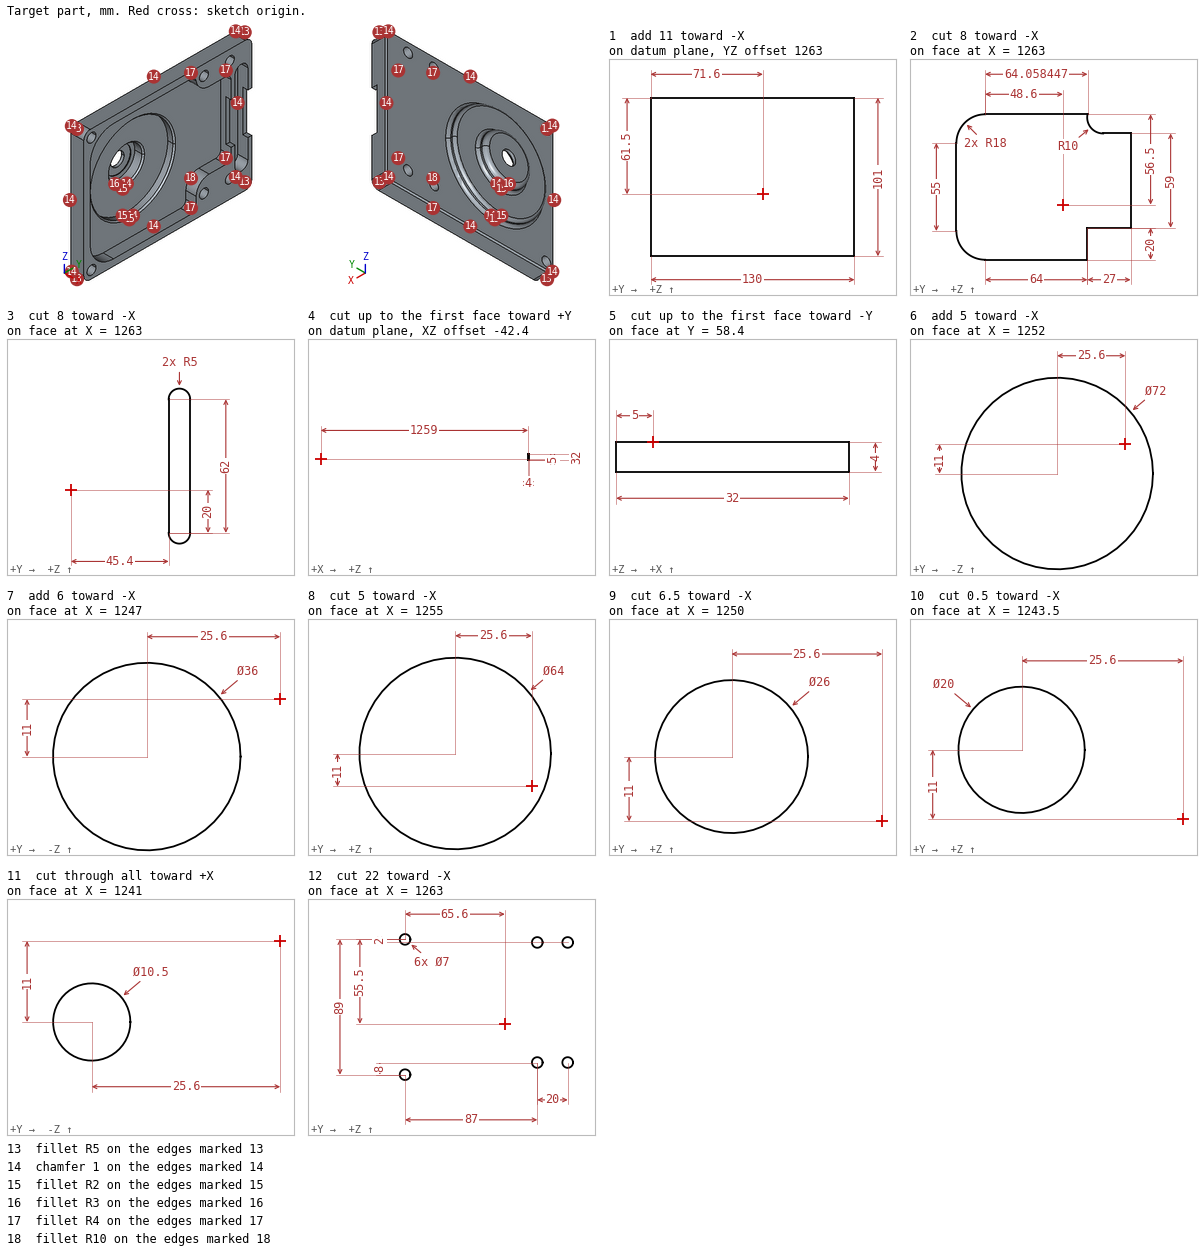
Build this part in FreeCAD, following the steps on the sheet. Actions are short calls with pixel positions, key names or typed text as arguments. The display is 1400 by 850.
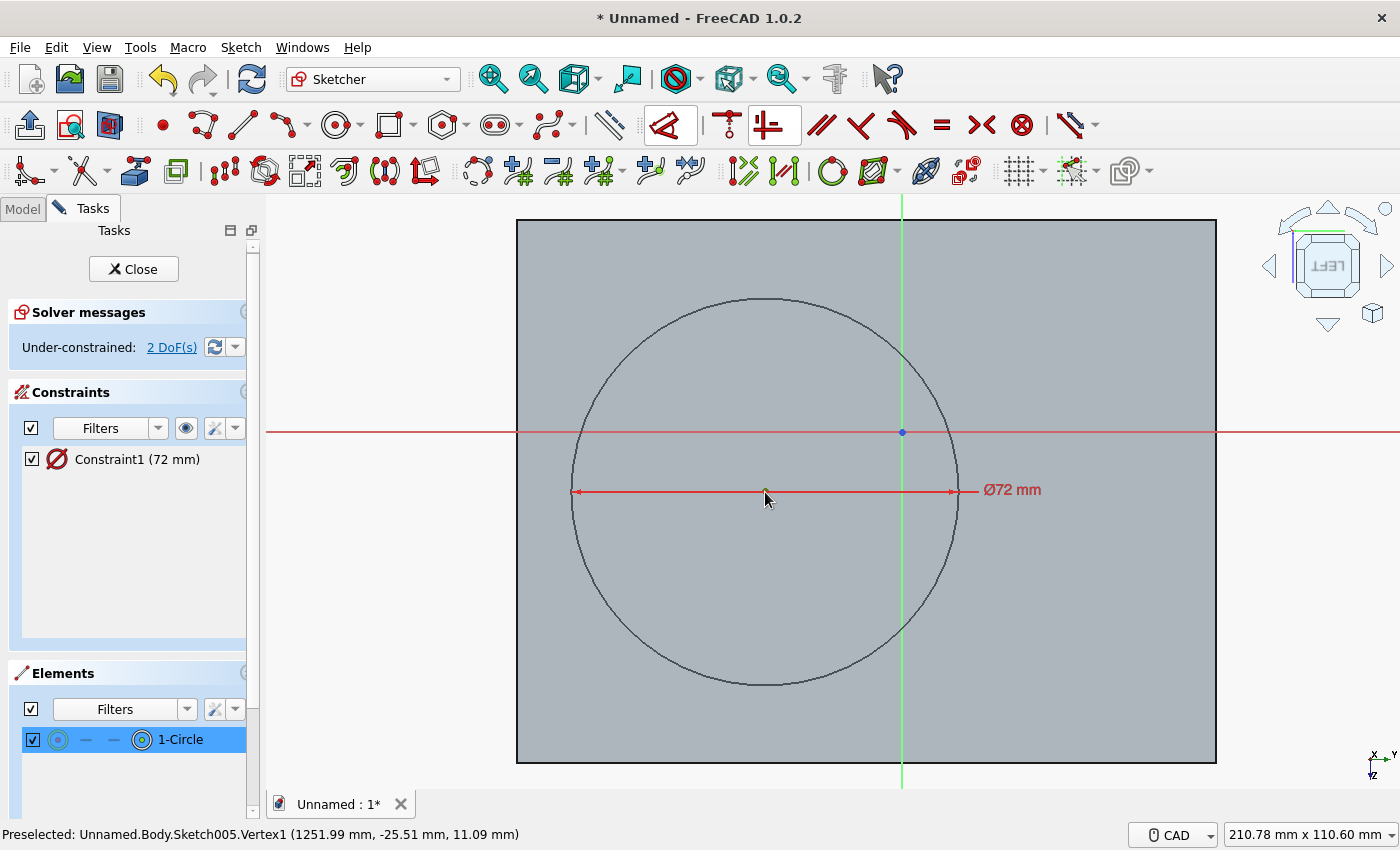
key(i)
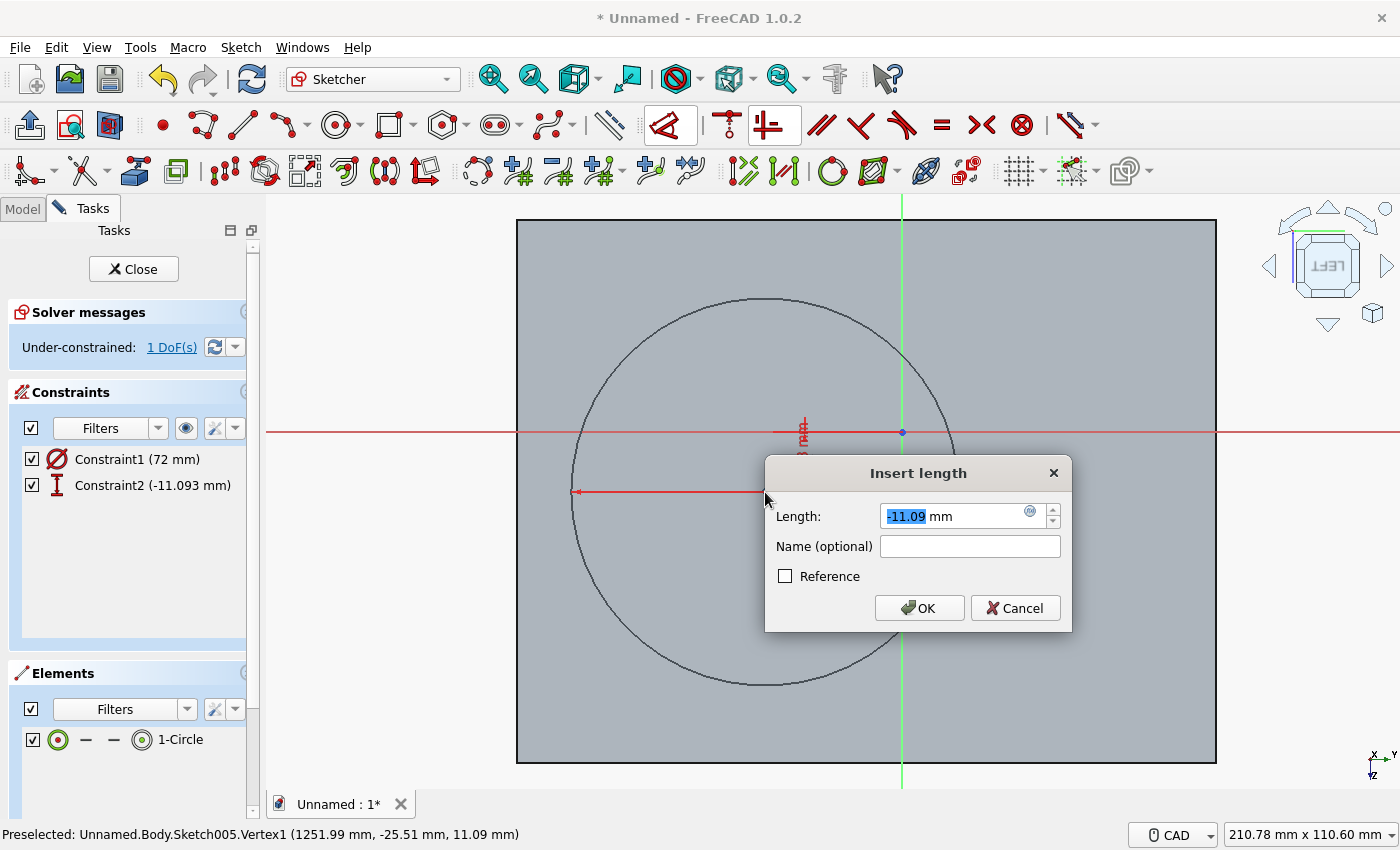
text(-11)
key(Return)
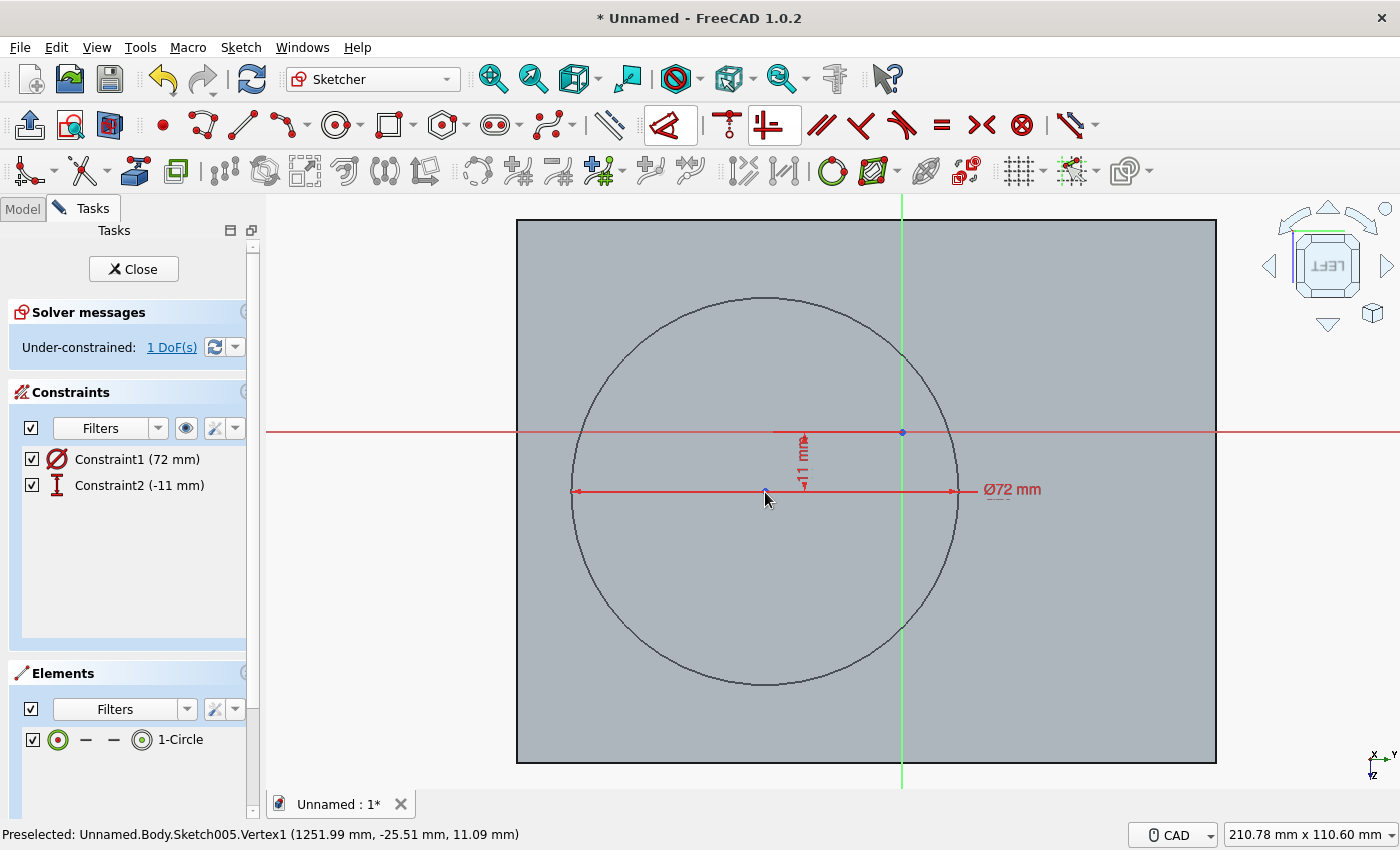
click(765, 491)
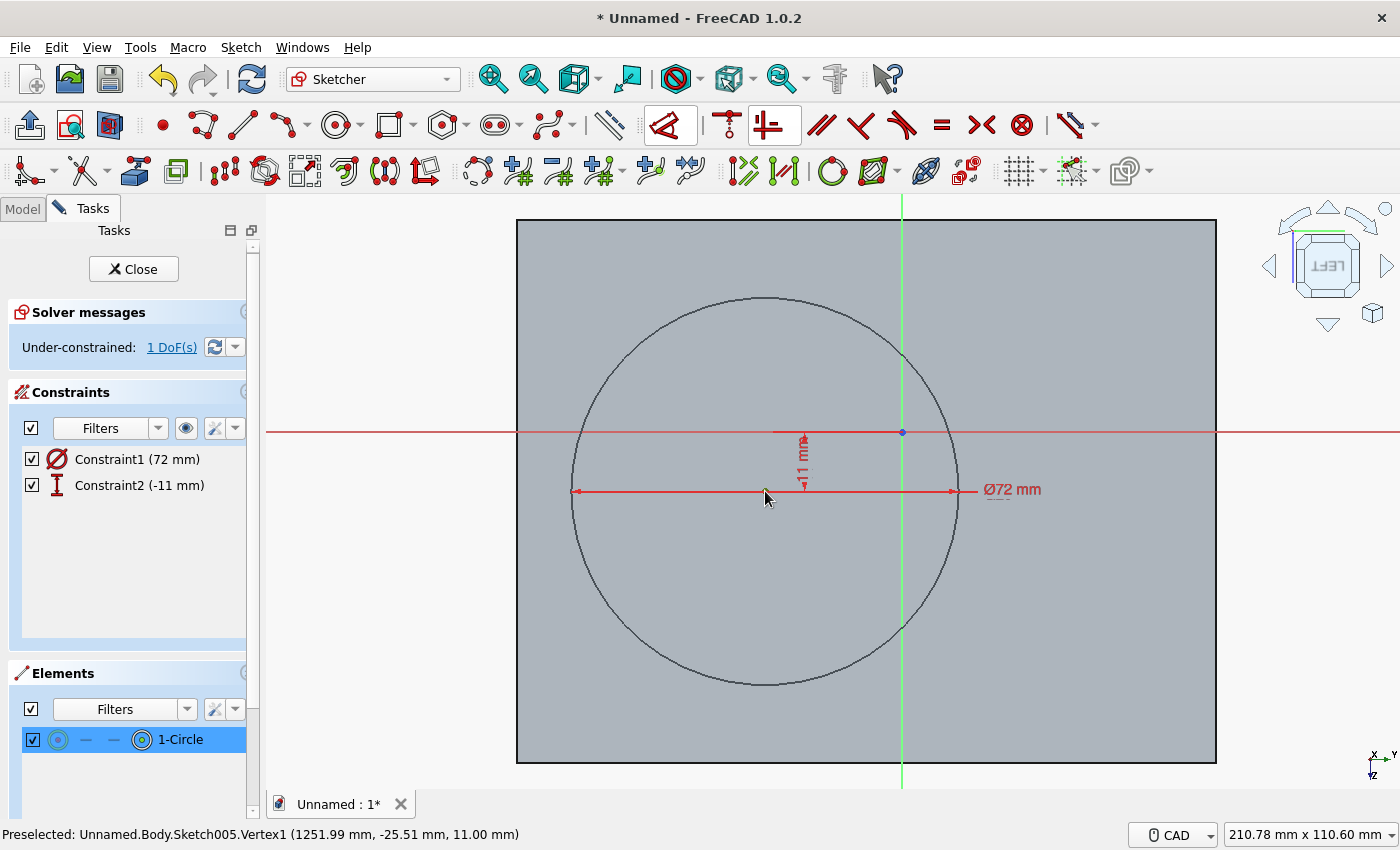
key(l)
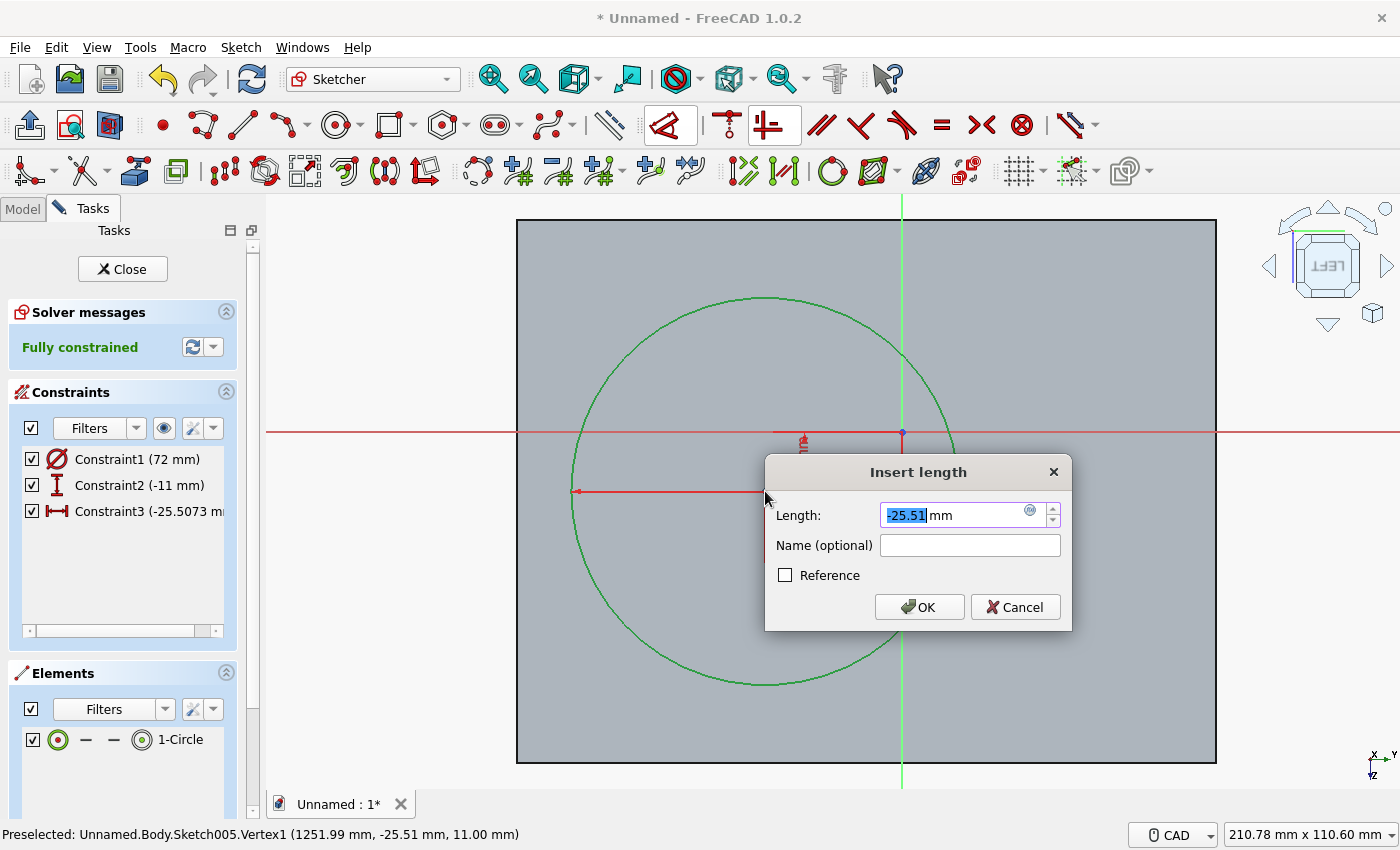
text(-25.6)
key(Return)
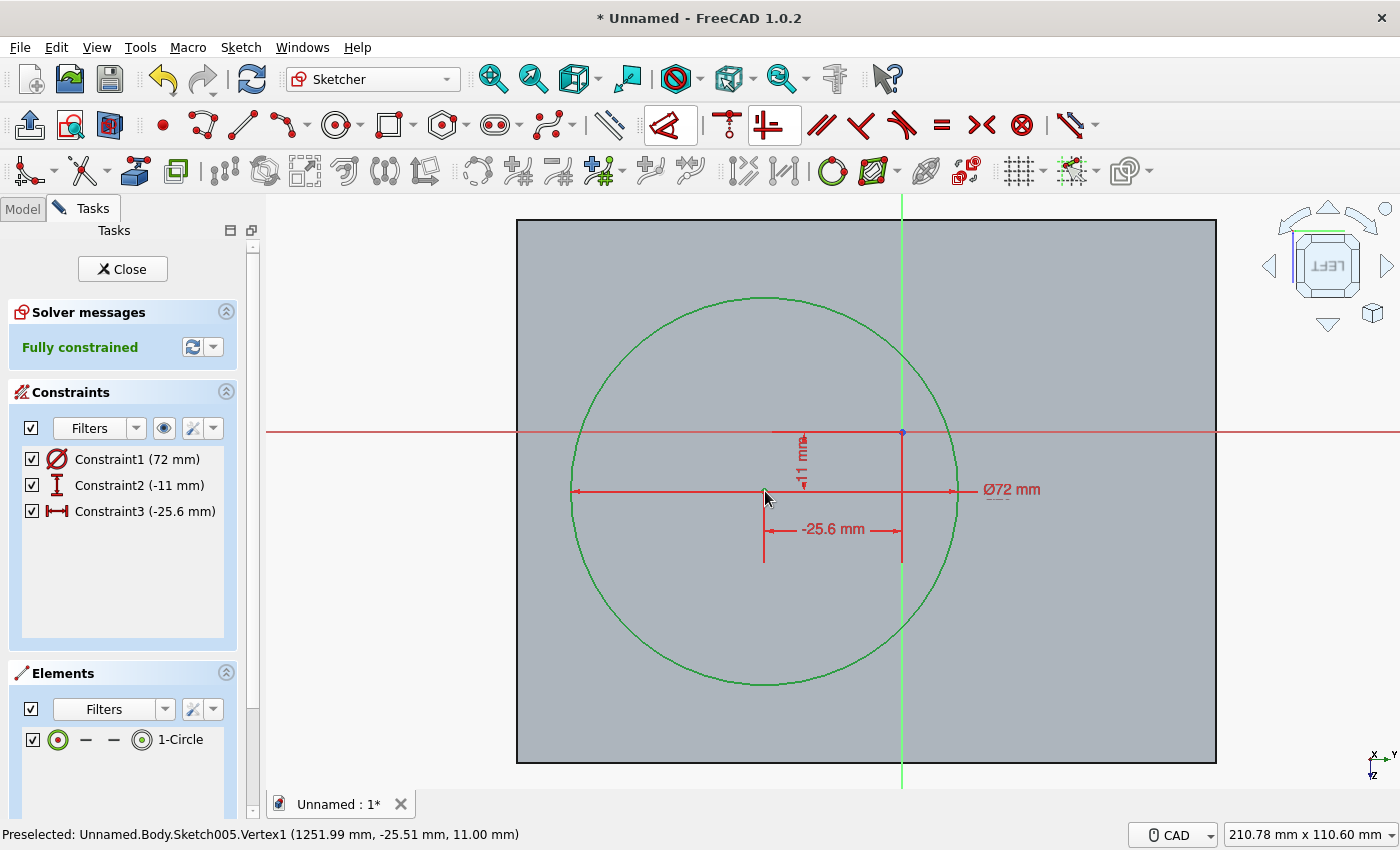
click(123, 269)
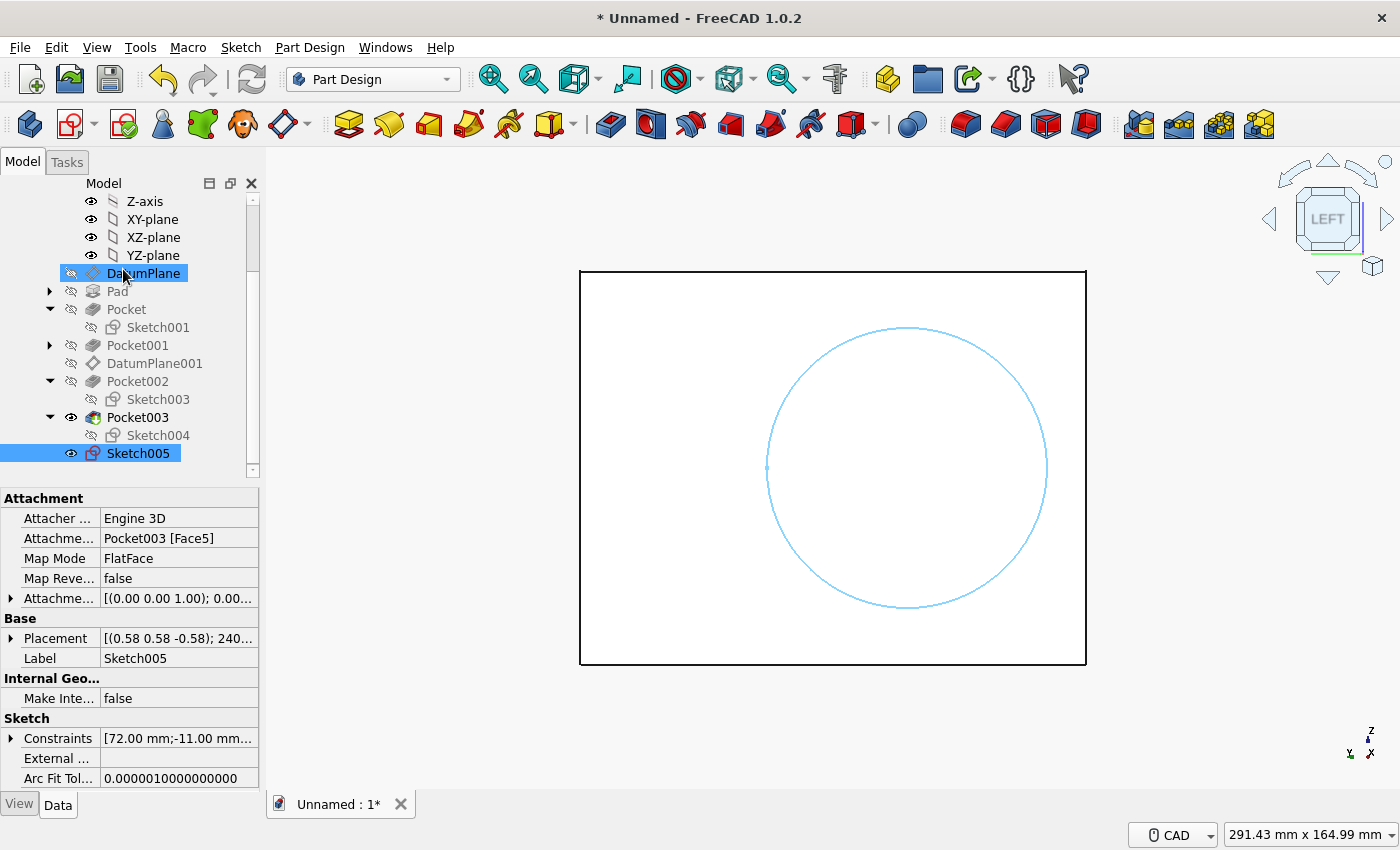
click(350, 124)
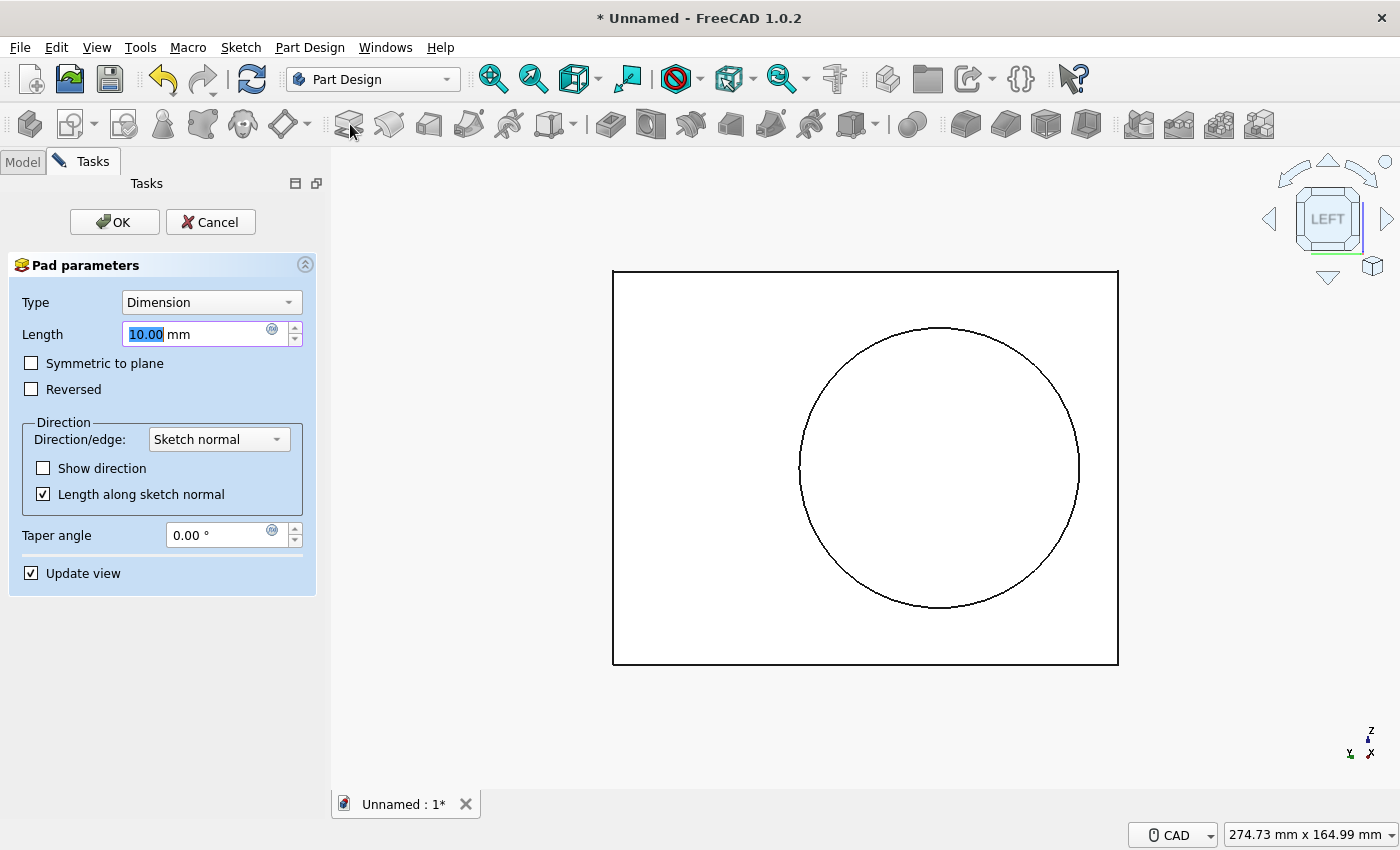
text(5)
key(Tab)